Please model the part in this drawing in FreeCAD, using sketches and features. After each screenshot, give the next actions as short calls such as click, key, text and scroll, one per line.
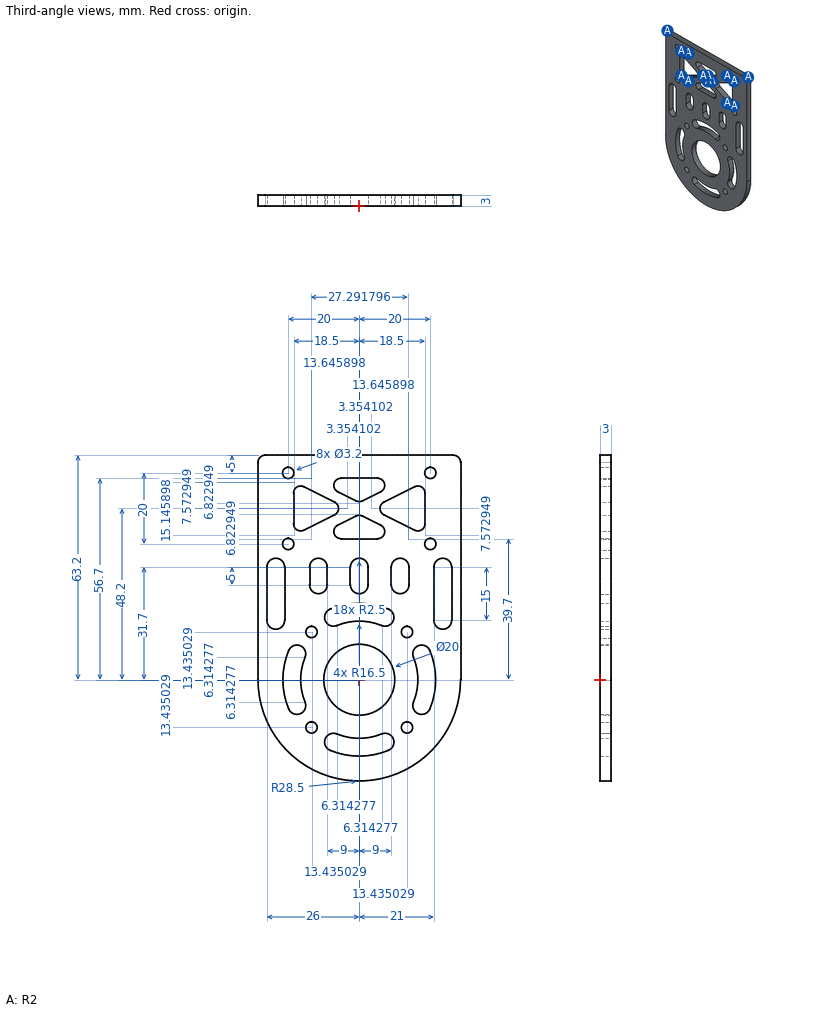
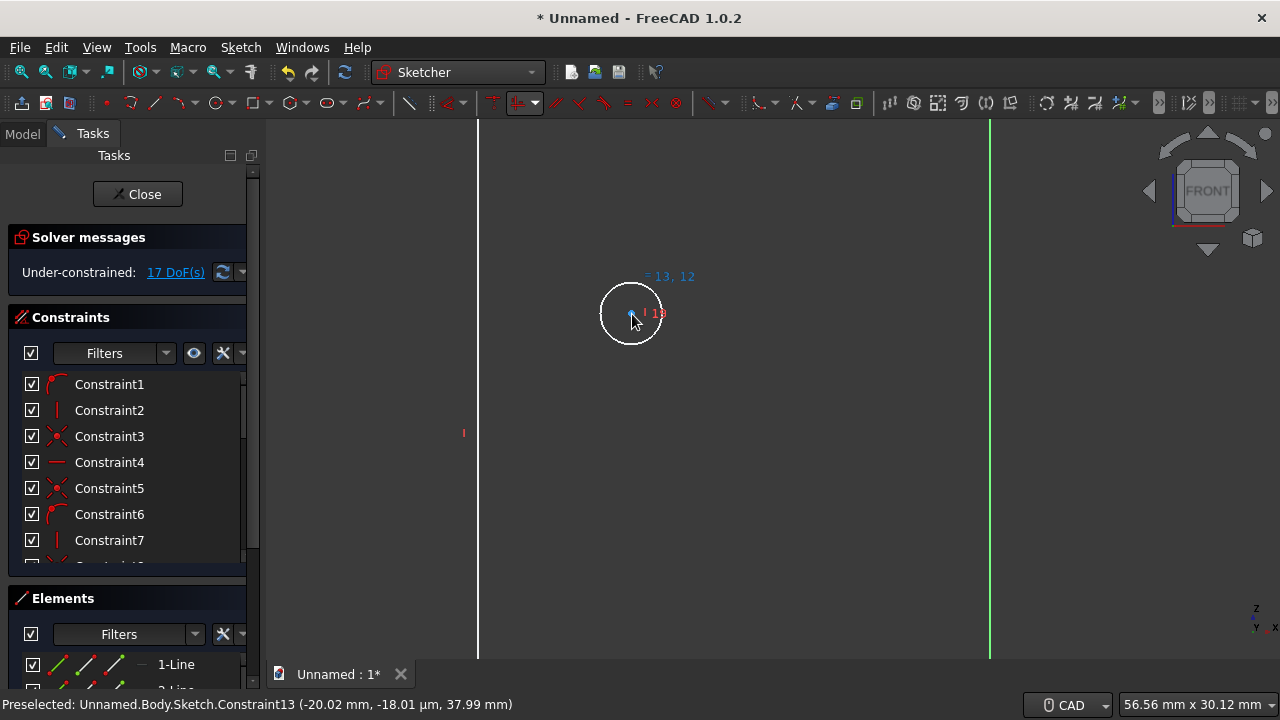
click(631, 313)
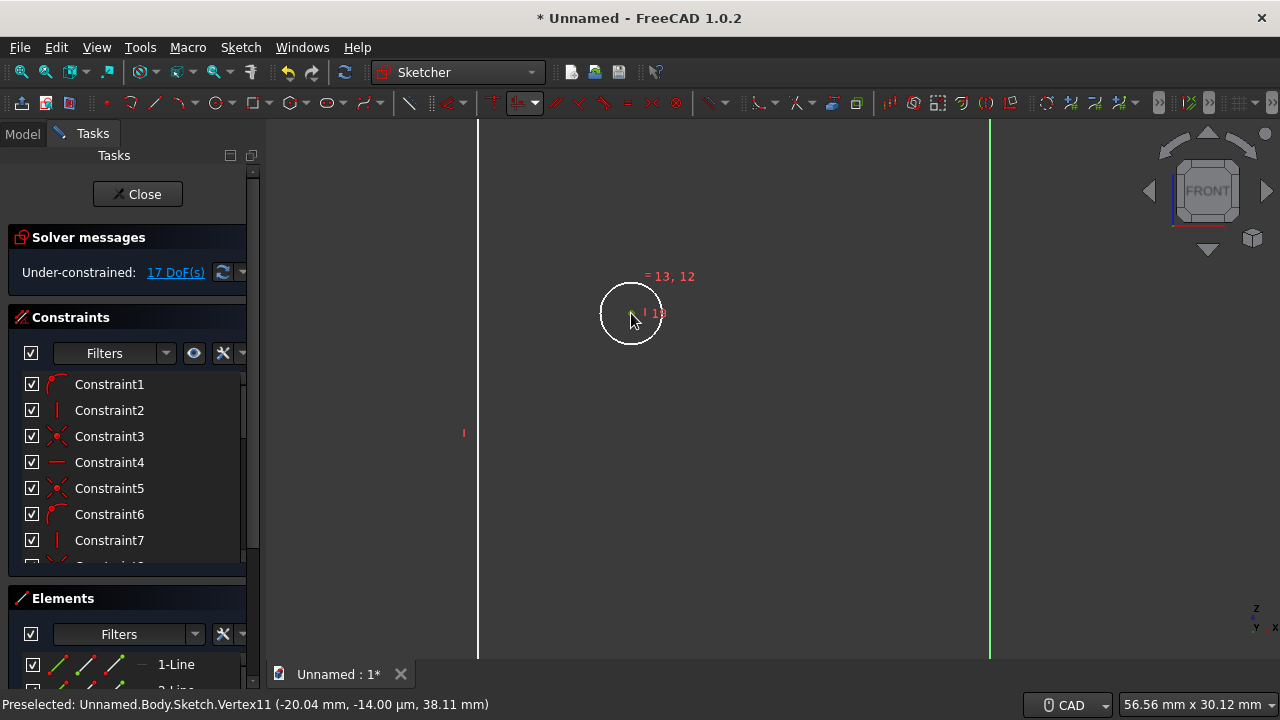
scroll(632, 314, down, 8)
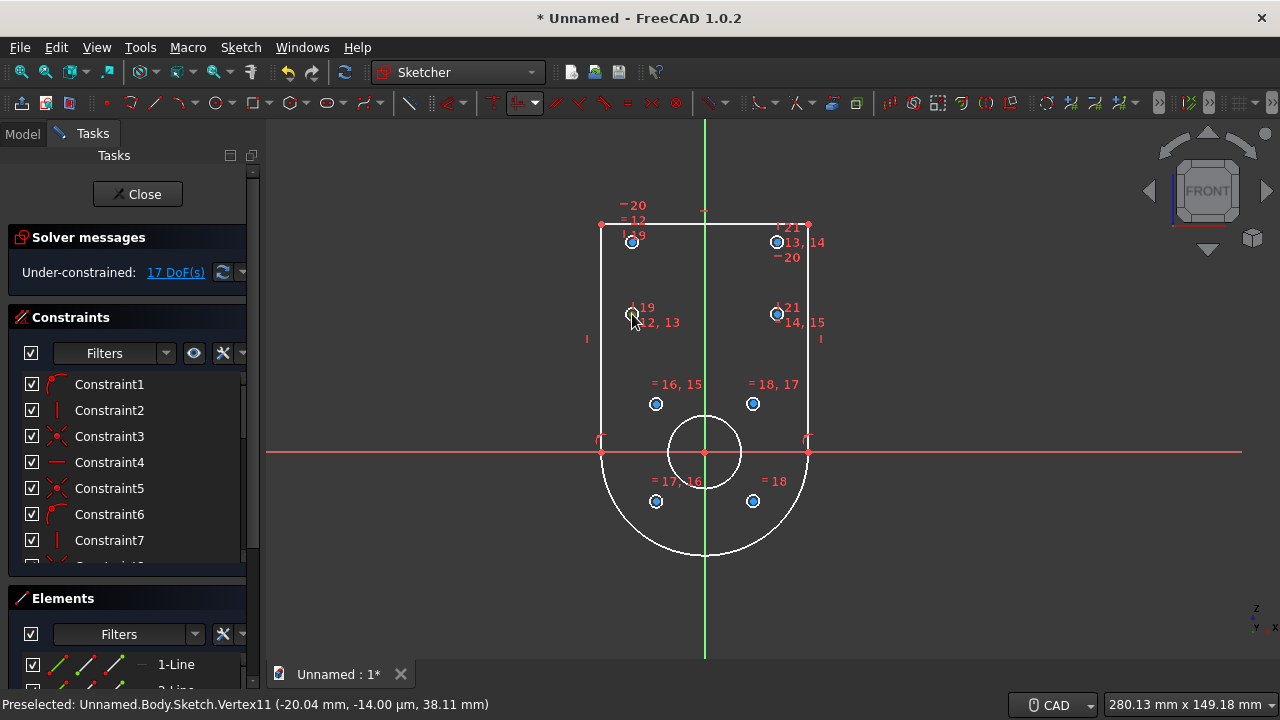
scroll(777, 314, up, 4)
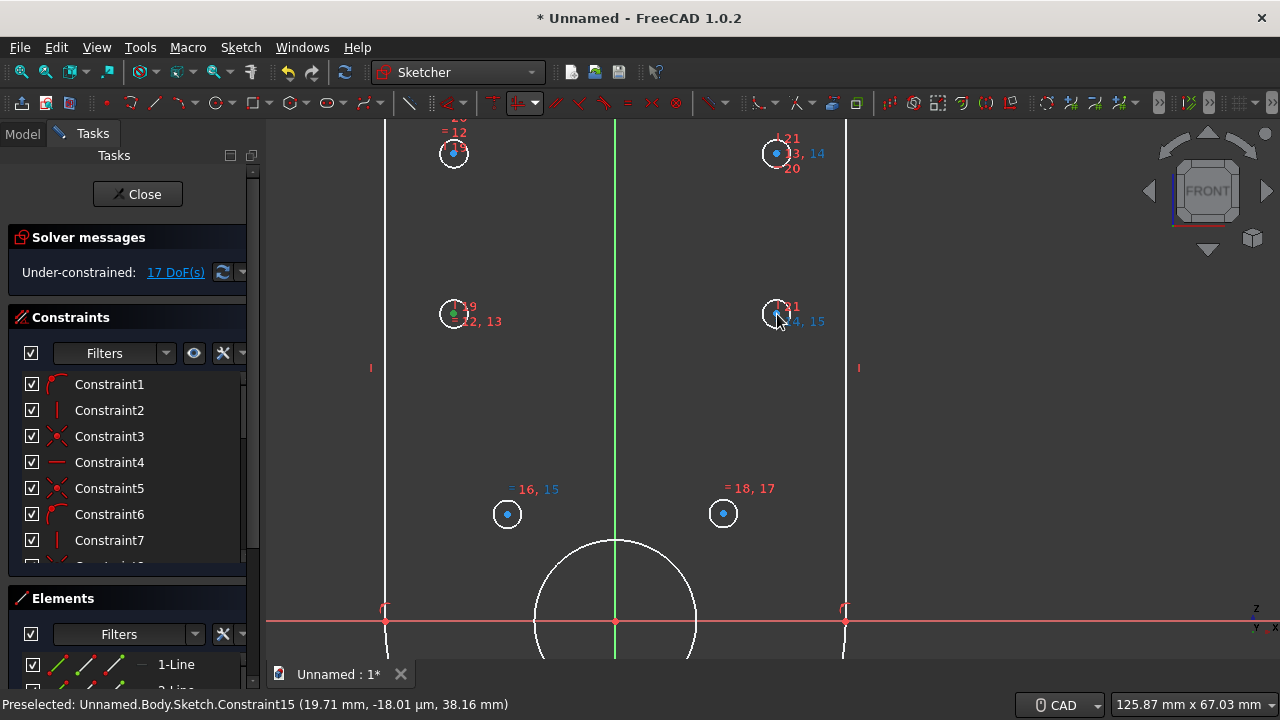
scroll(777, 314, up, 4)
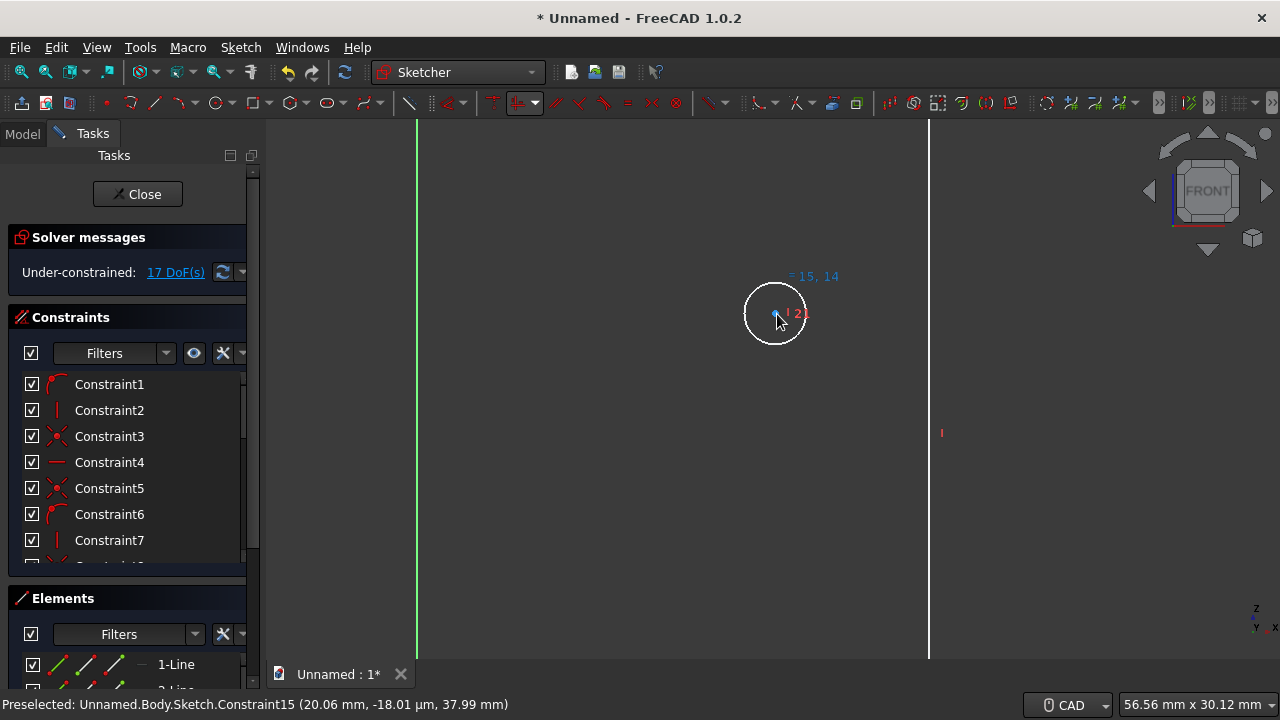
click(775, 313)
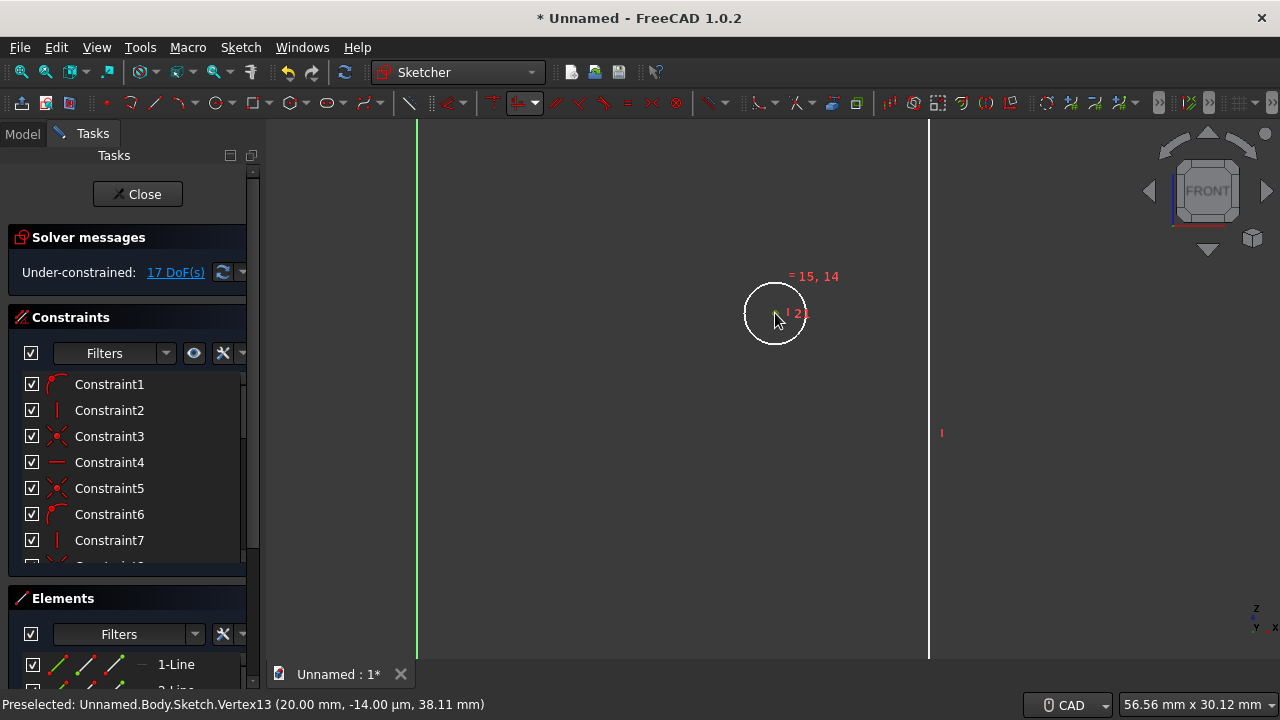
key(h)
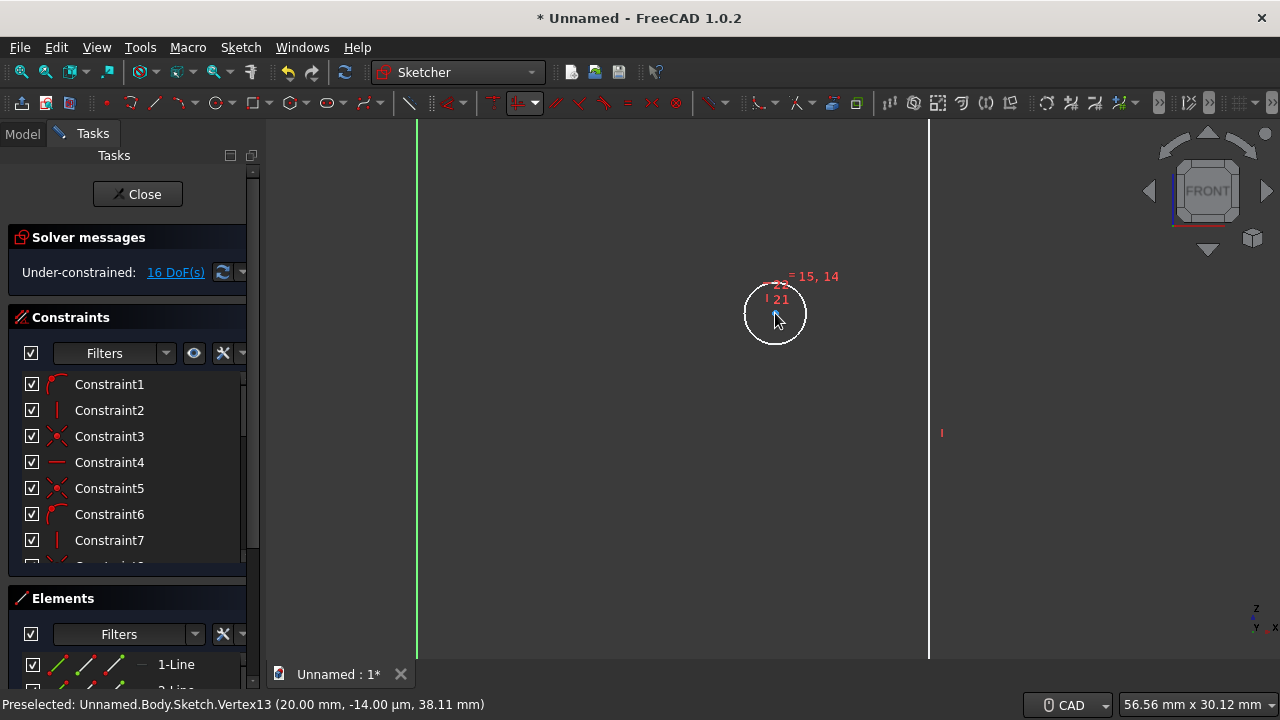
scroll(777, 314, down, 8)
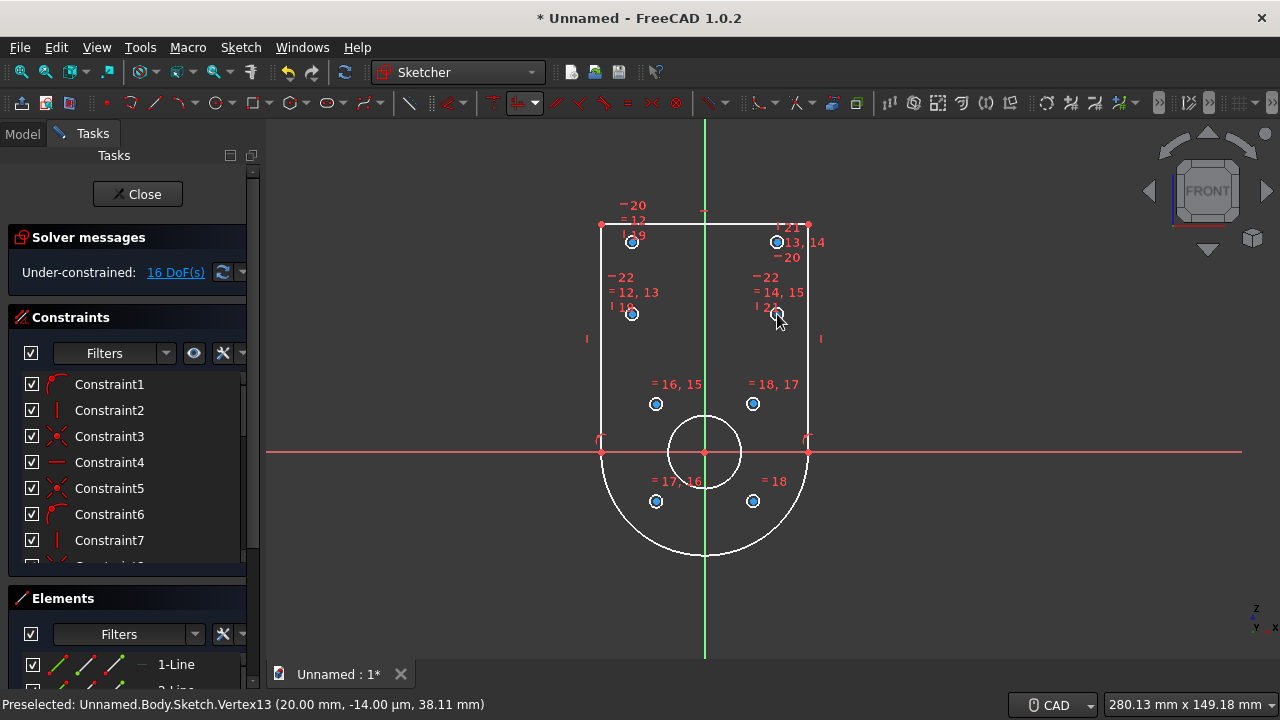
click(656, 404)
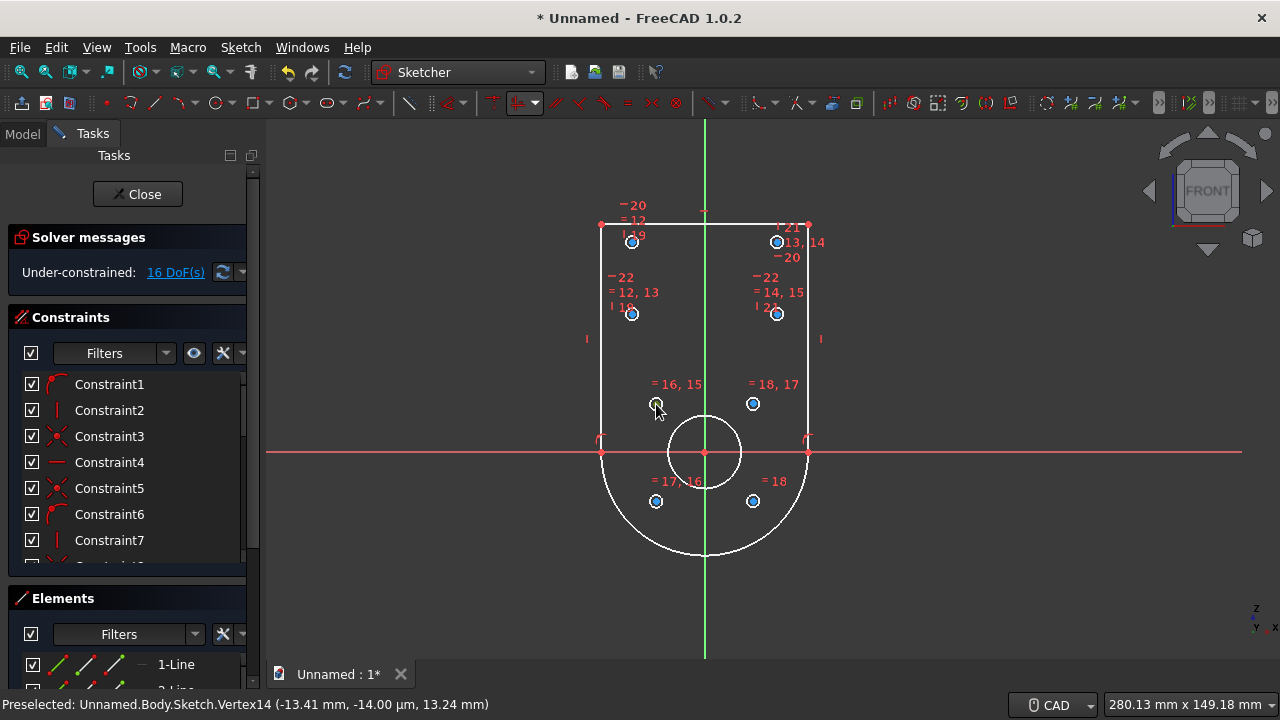
click(656, 501)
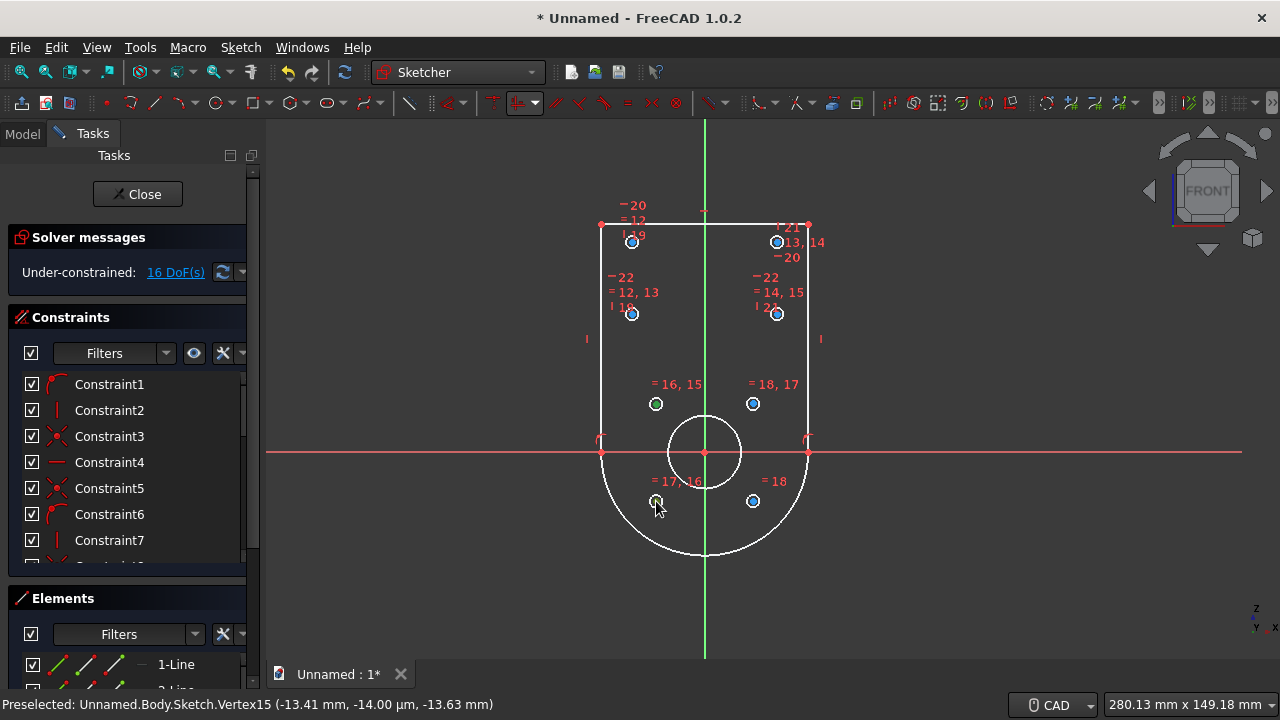
key(v)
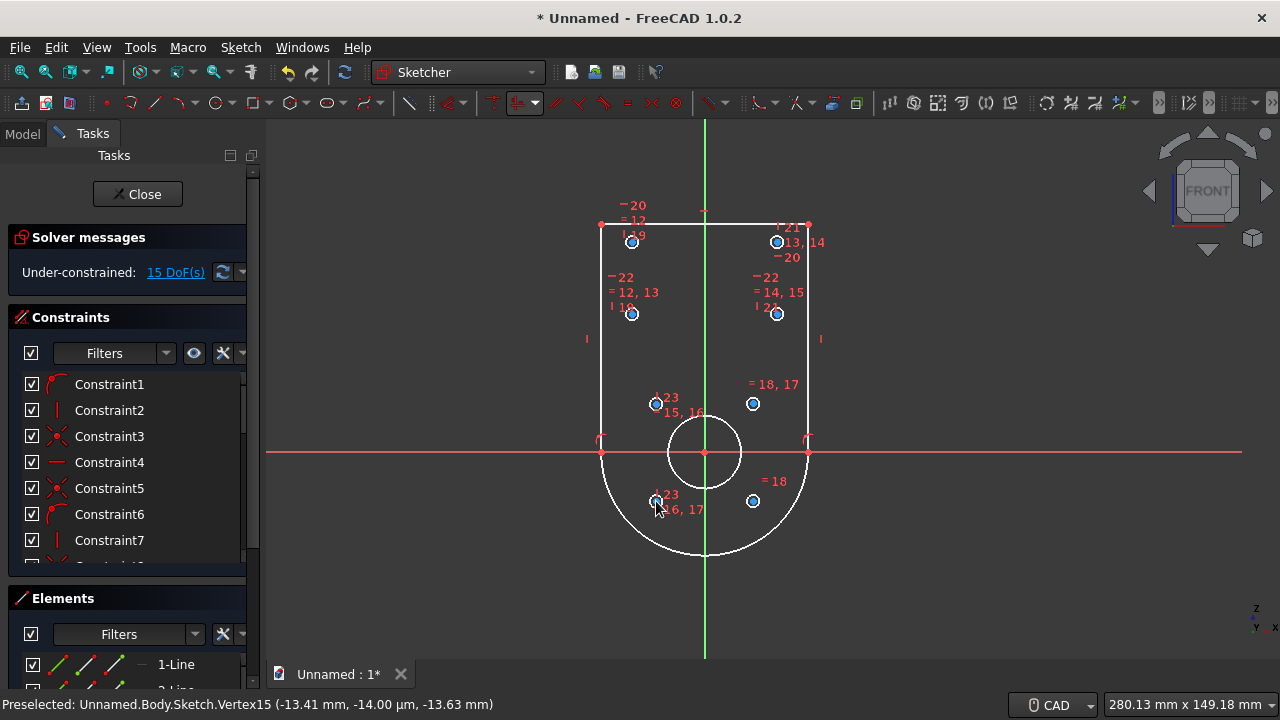
click(656, 404)